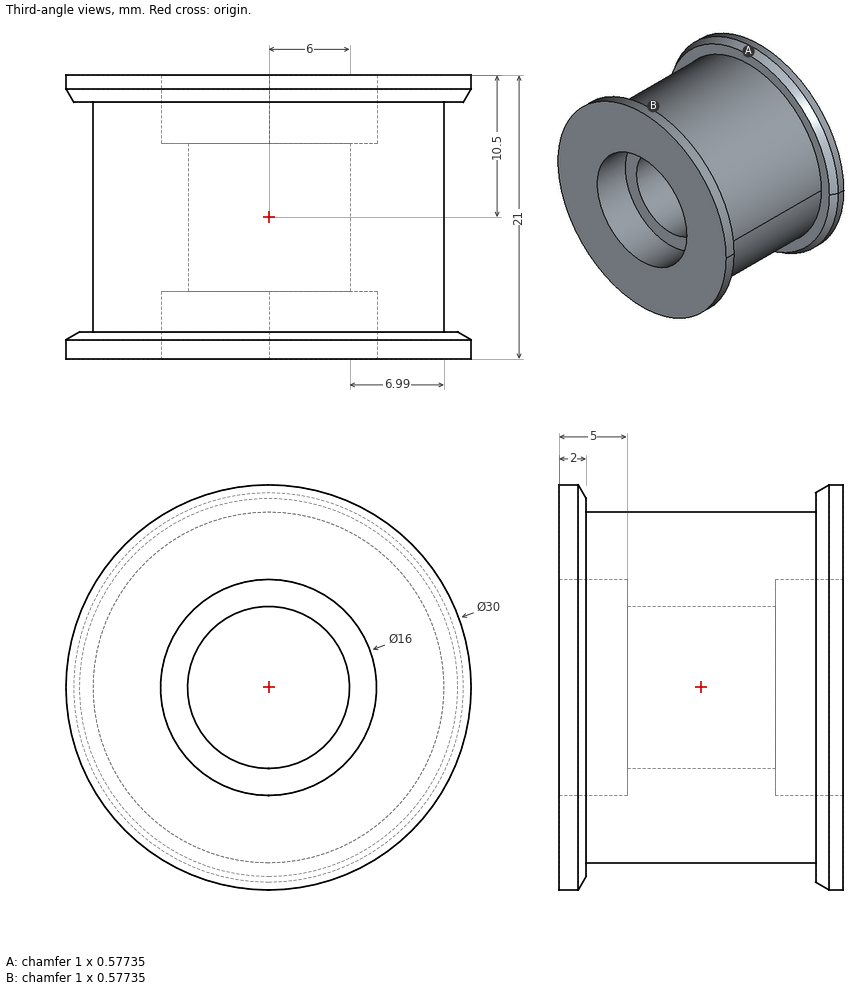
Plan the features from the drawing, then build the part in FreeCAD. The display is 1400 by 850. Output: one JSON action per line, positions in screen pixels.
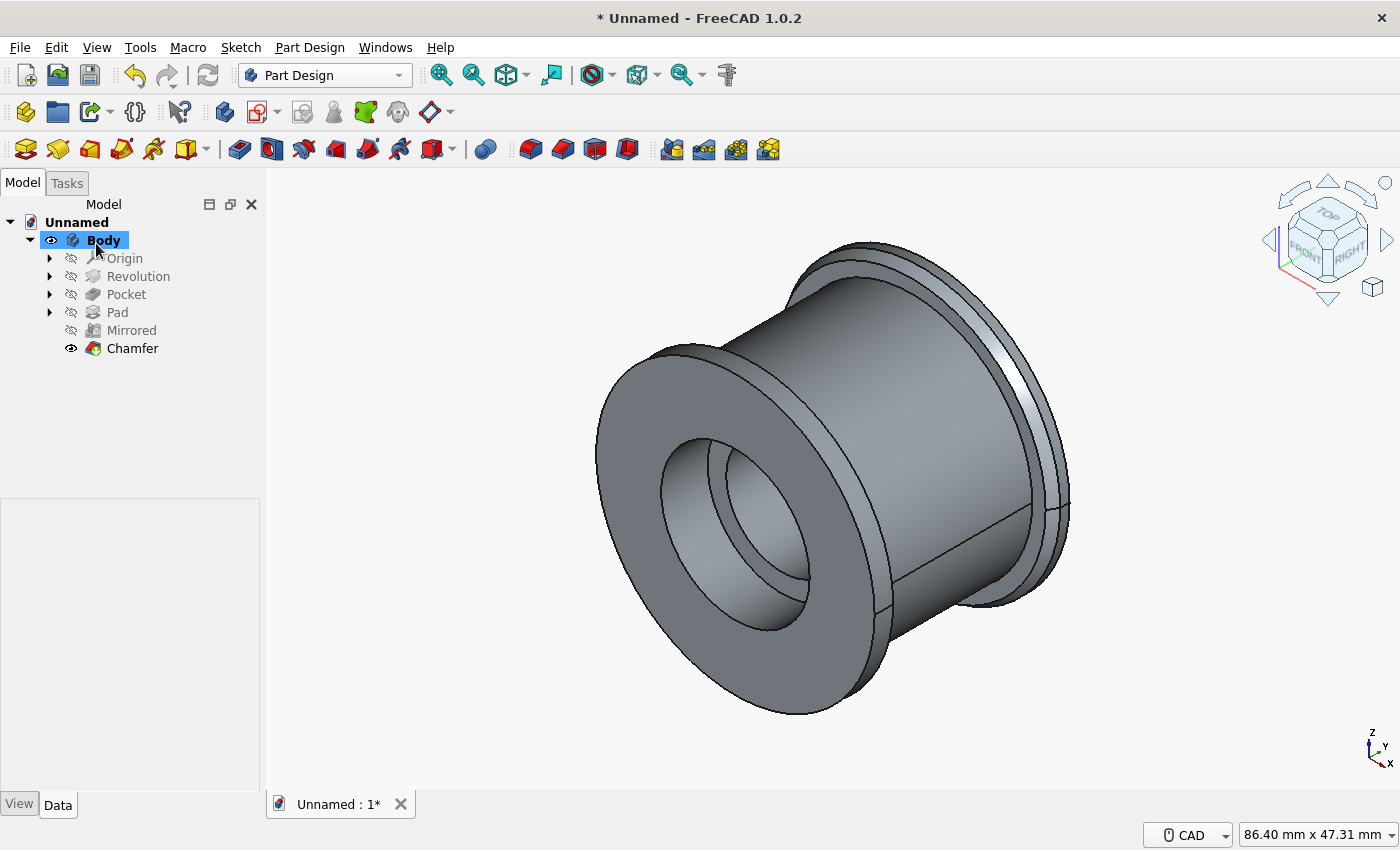
{"action": "key", "text": "2"}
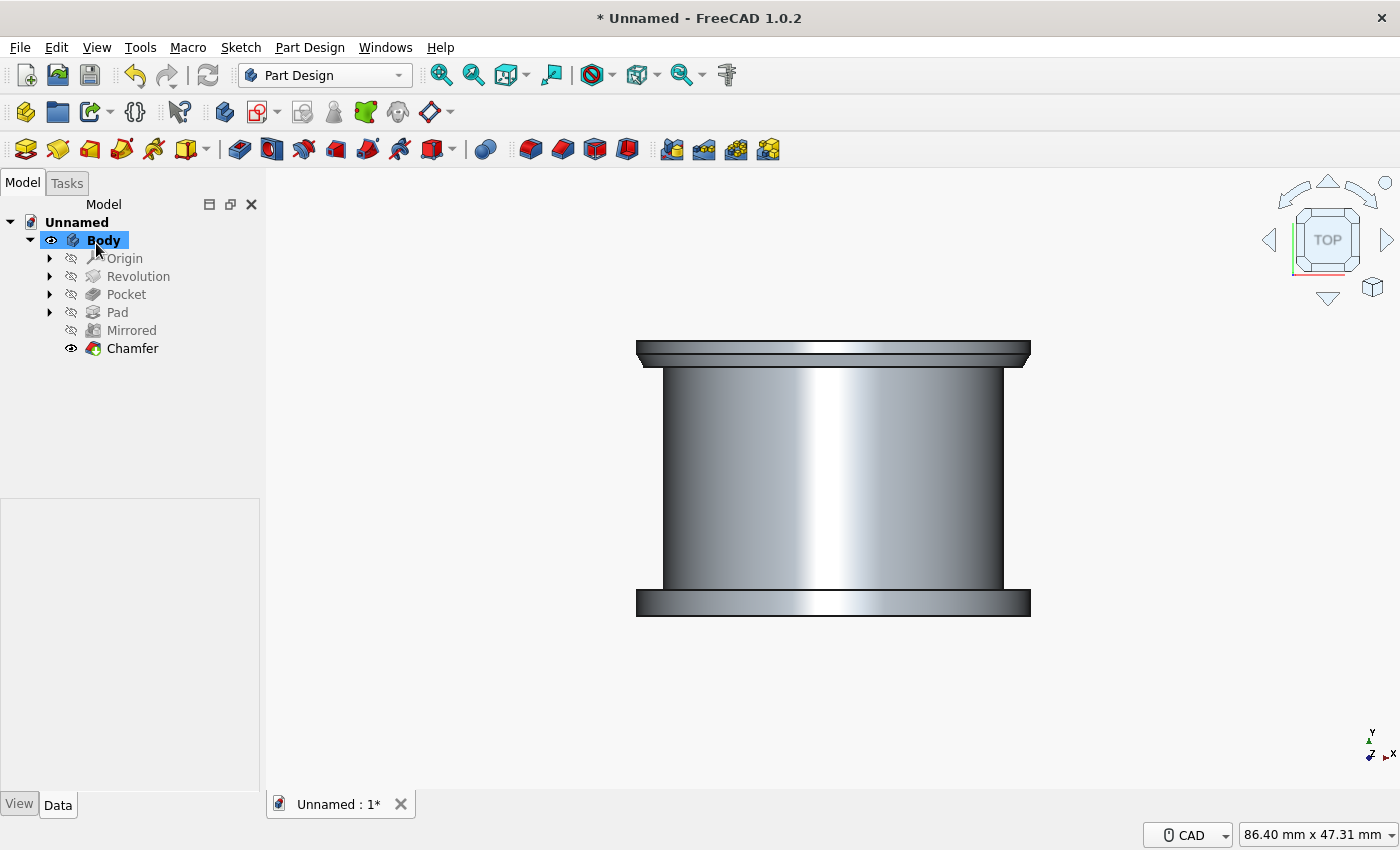
{"action": "left_click", "coordinate": [442, 76]}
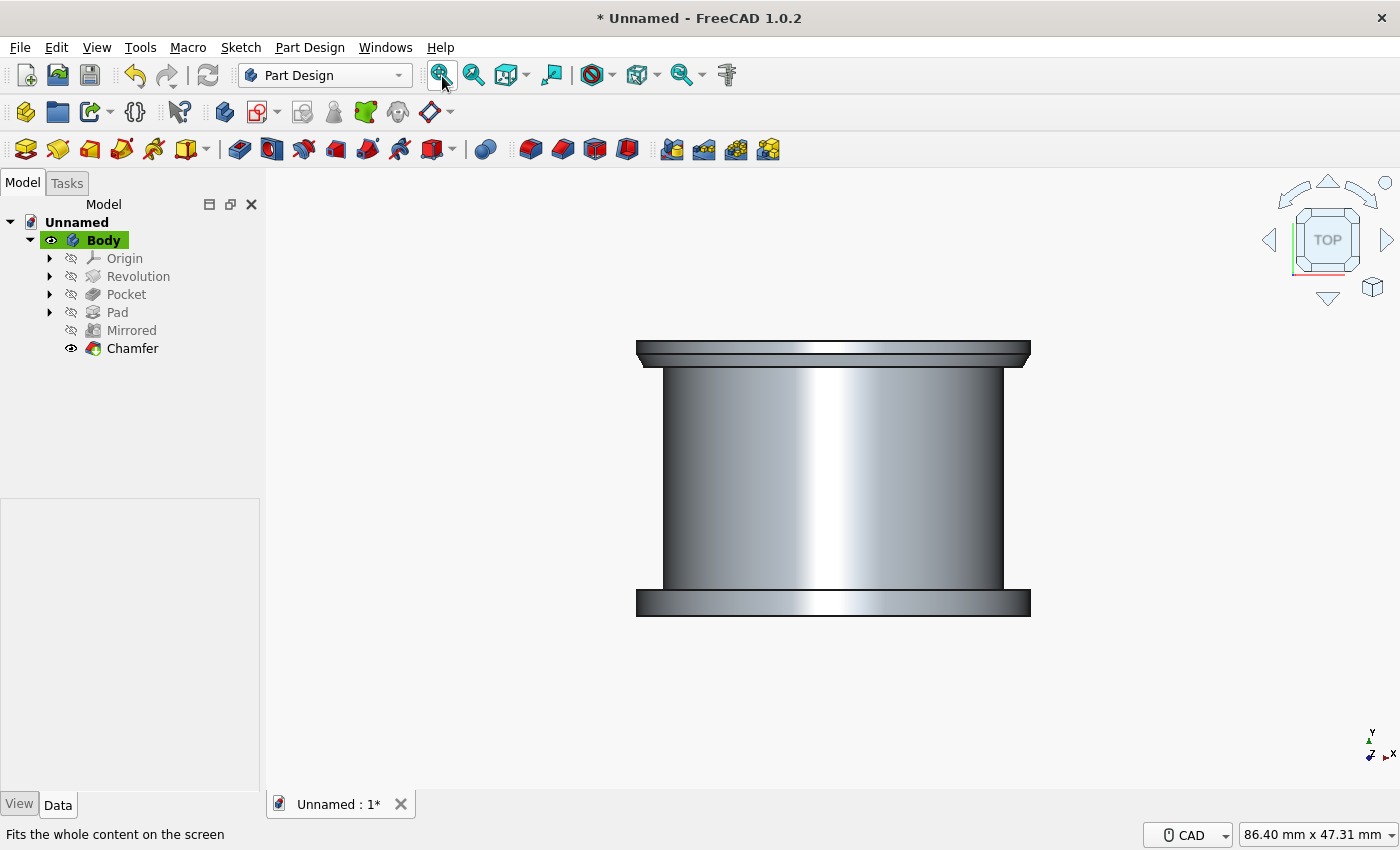
{"action": "left_click", "coordinate": [674, 589]}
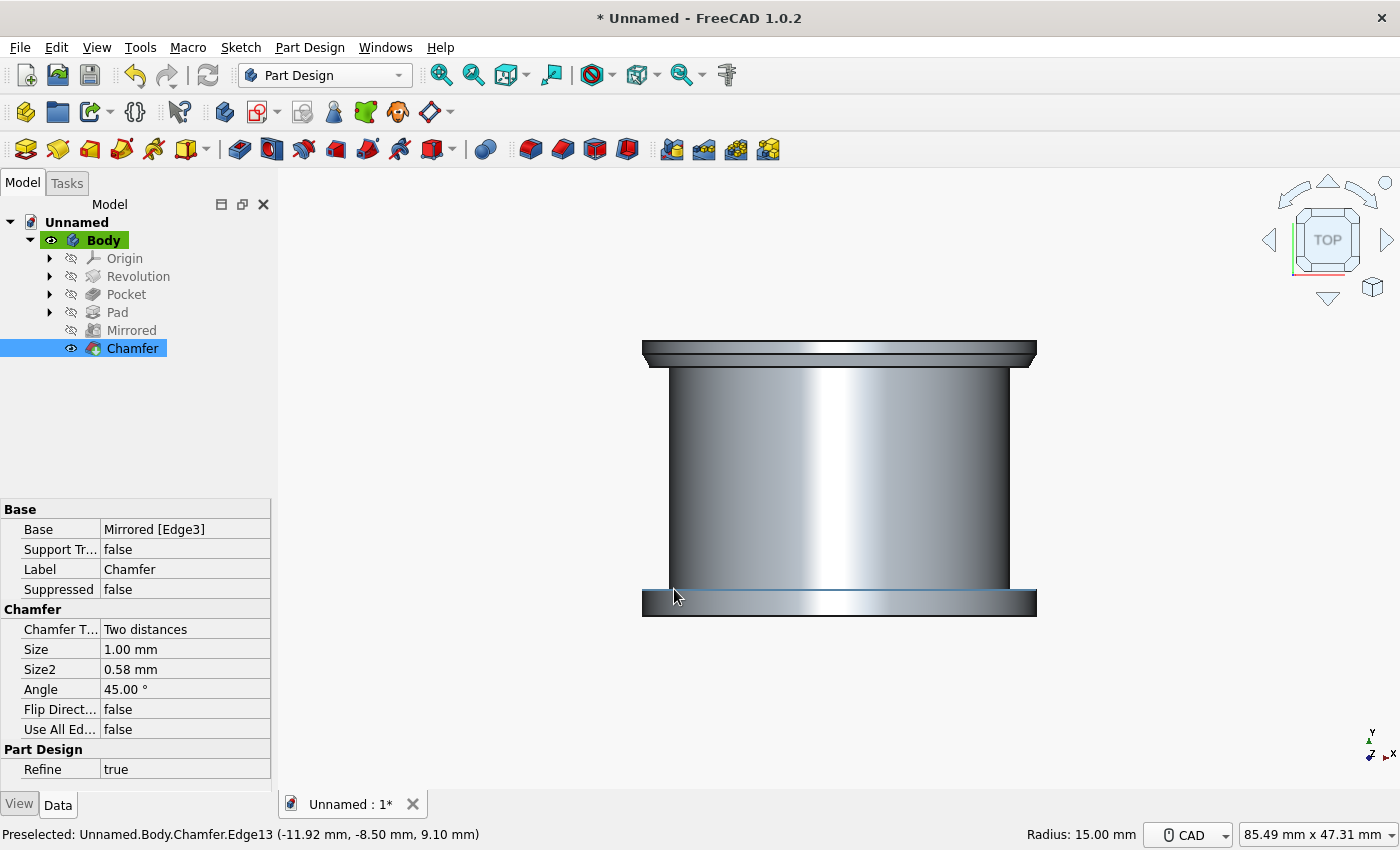
{"action": "left_click", "coordinate": [564, 150]}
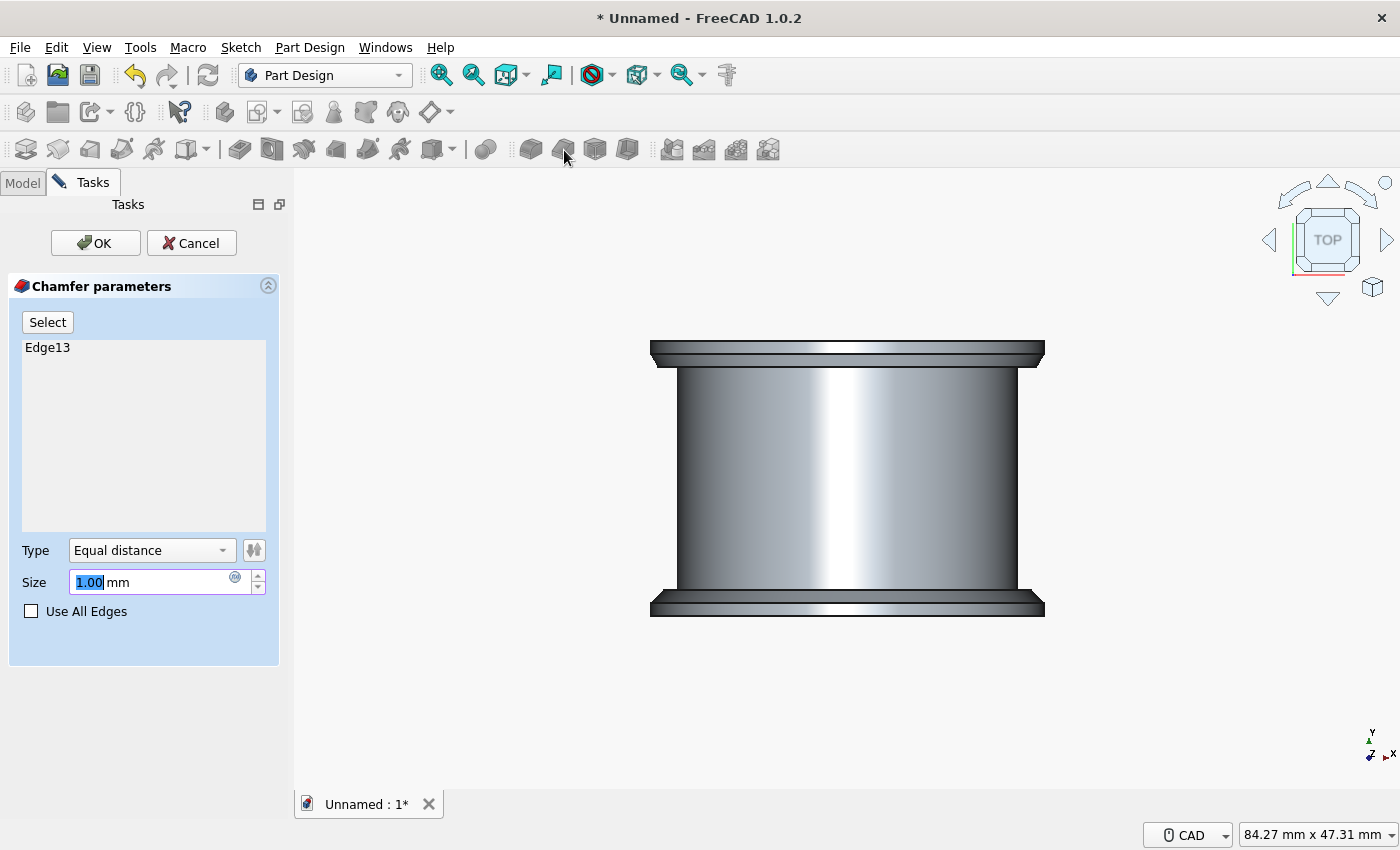
{"action": "type", "text": "1"}
{"action": "key", "text": "Tab"}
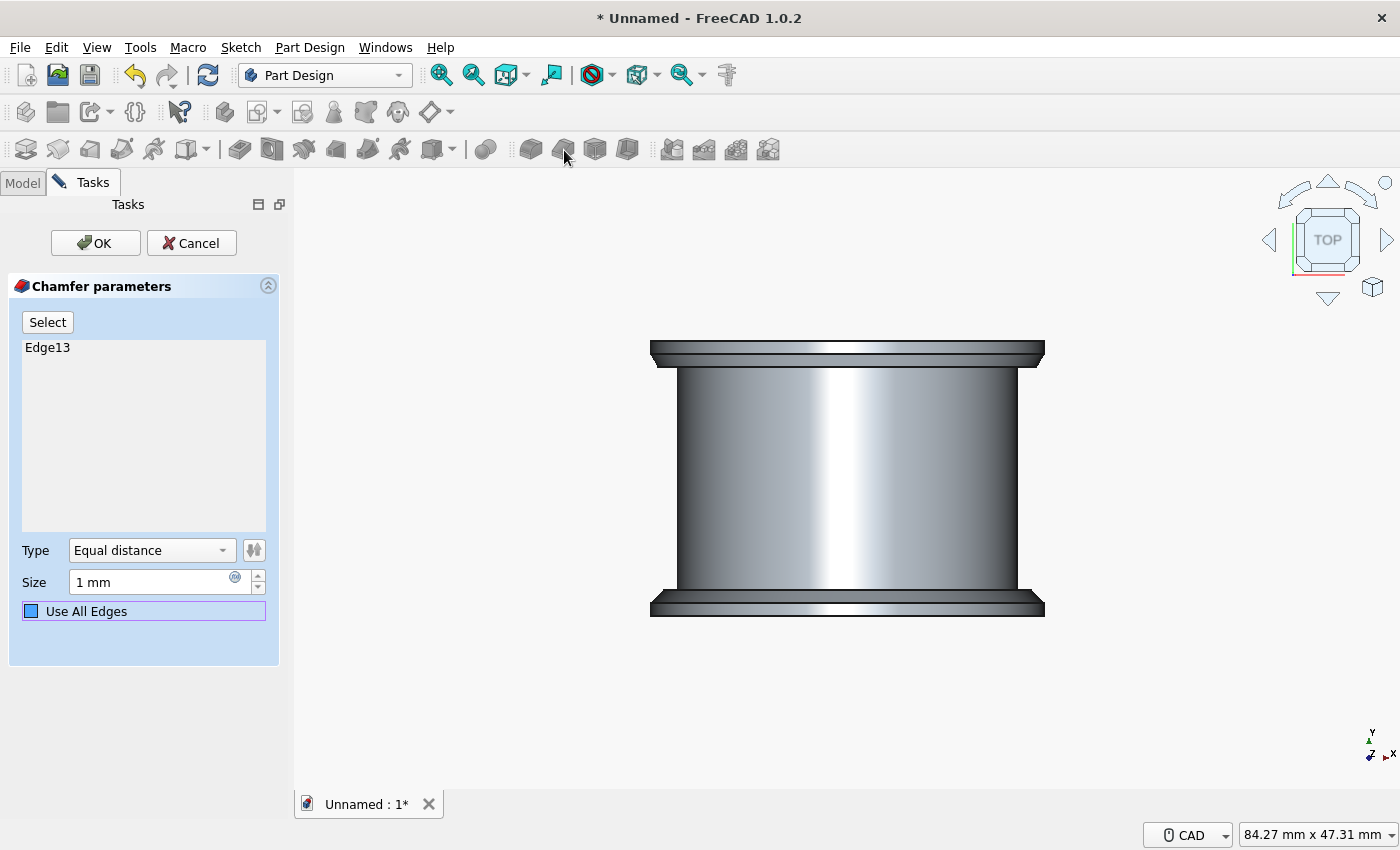
{"action": "left_click", "coordinate": [153, 550]}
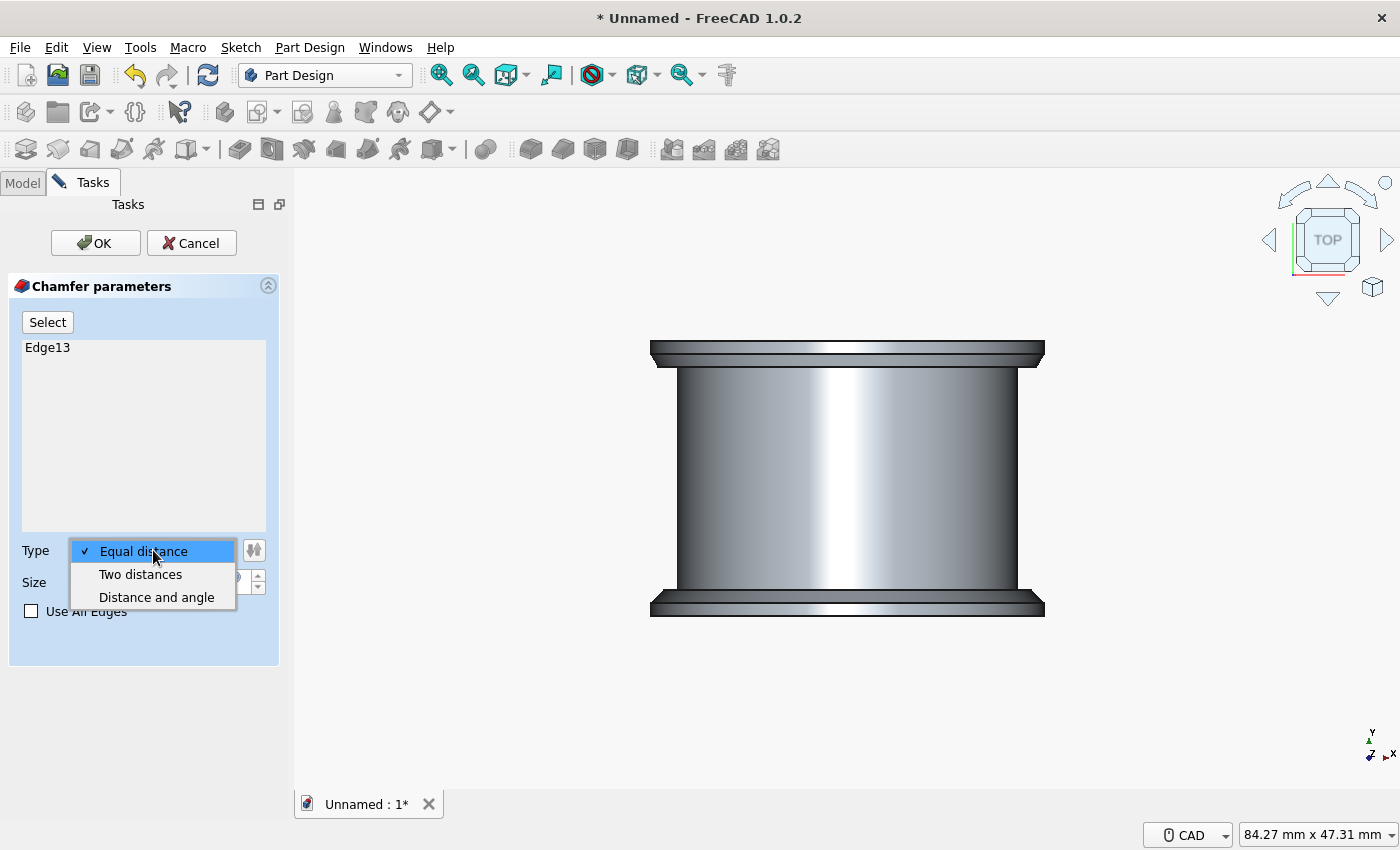
{"action": "left_click", "coordinate": [152, 574]}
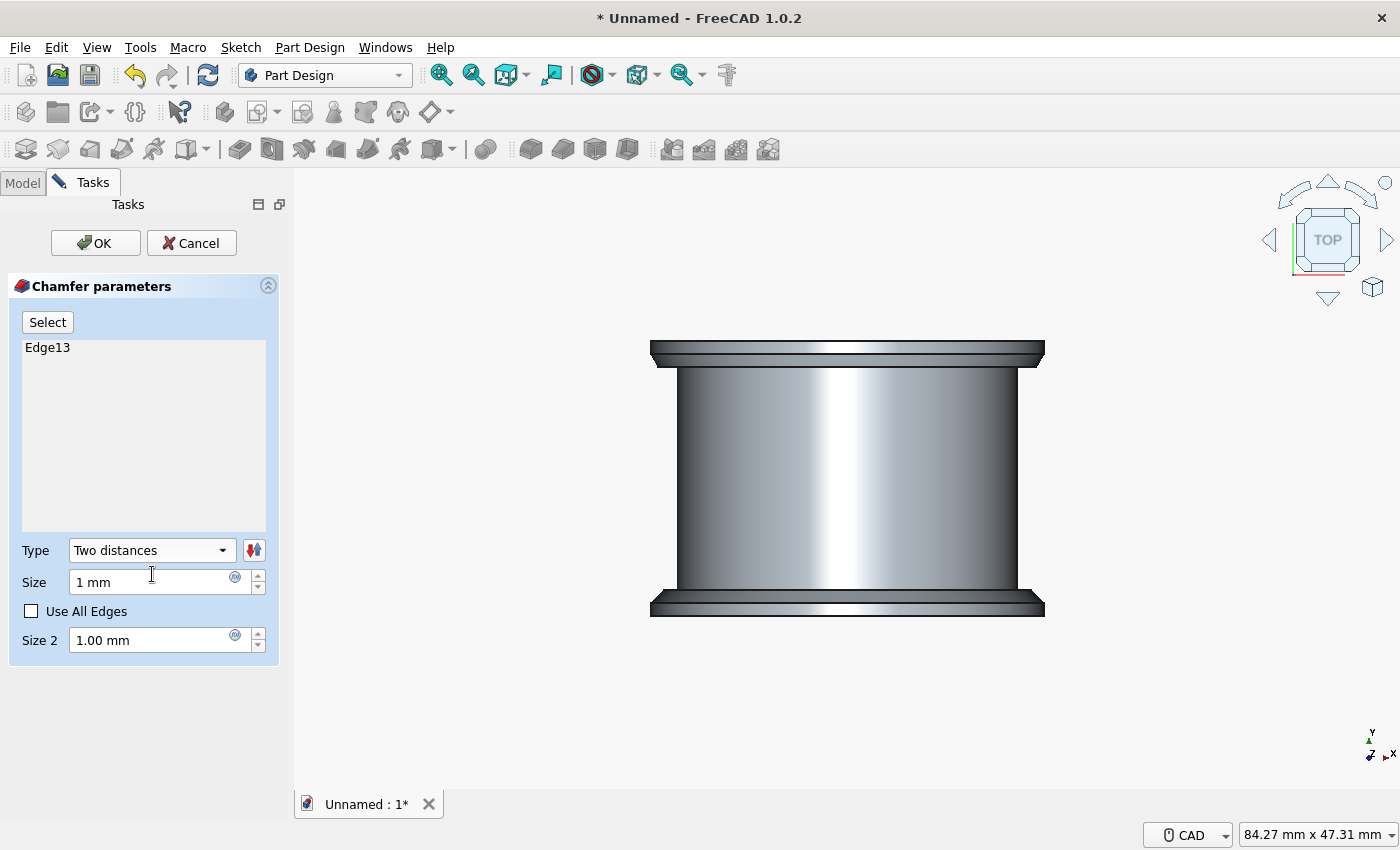
{"action": "triple_click", "coordinate": [160, 640]}